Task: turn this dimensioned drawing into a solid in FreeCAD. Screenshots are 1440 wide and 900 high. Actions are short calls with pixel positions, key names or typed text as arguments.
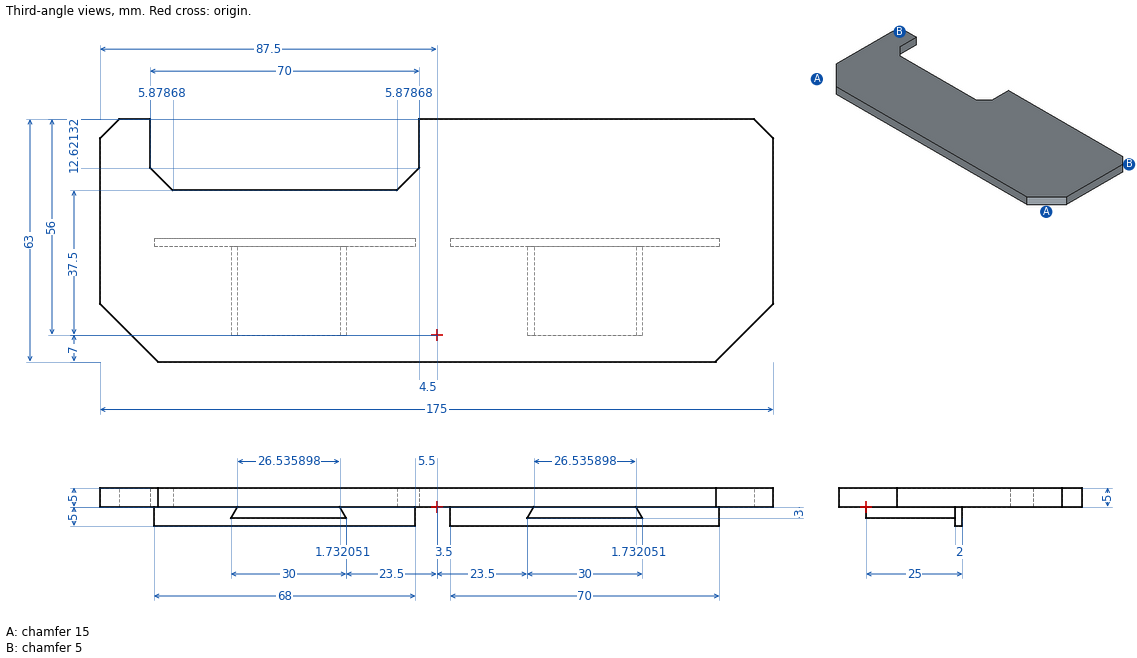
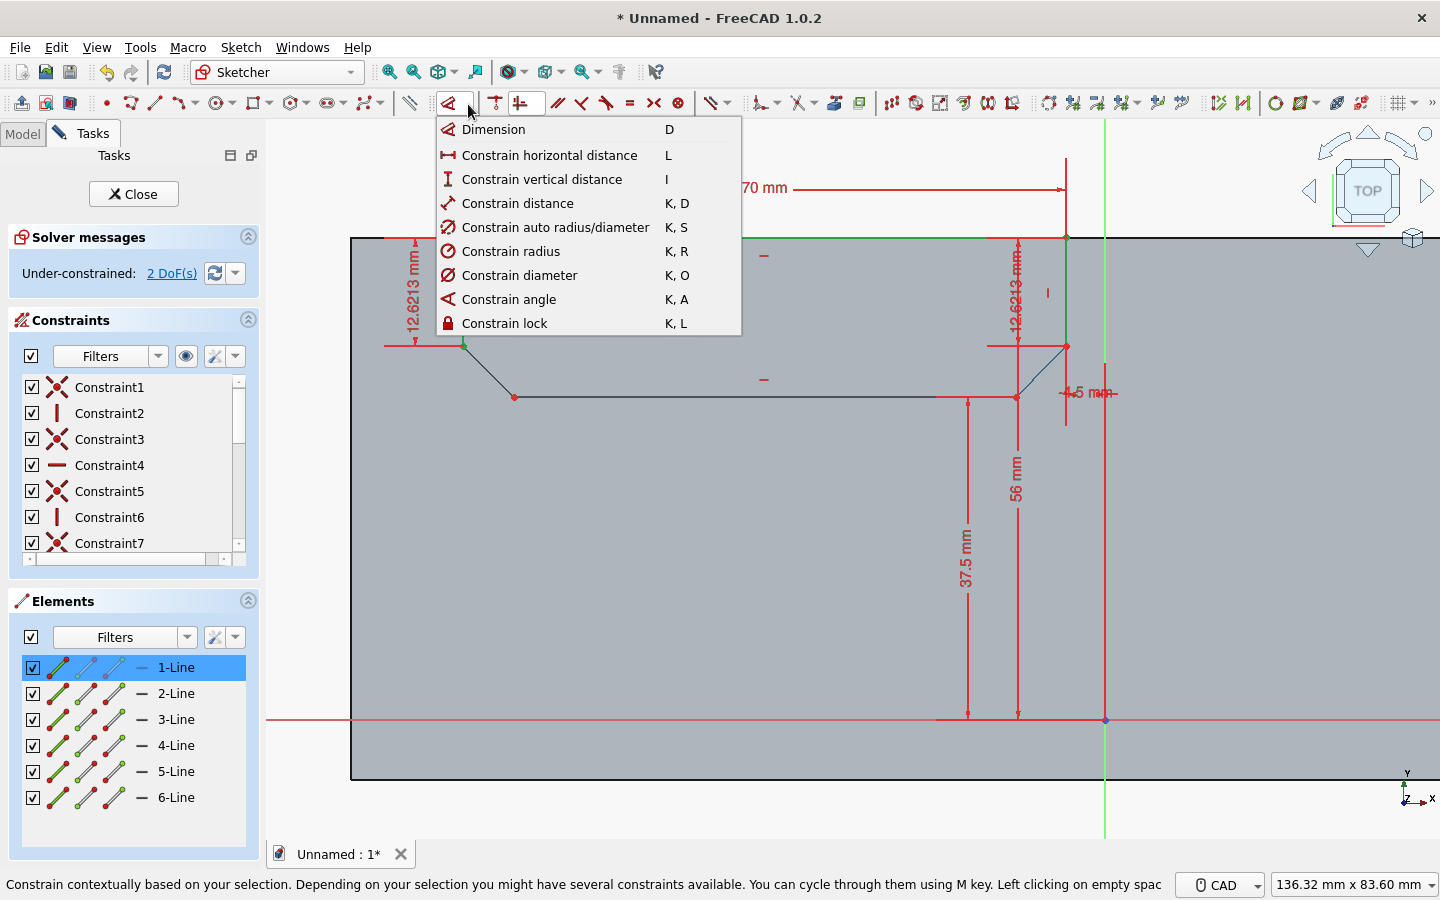
click(589, 155)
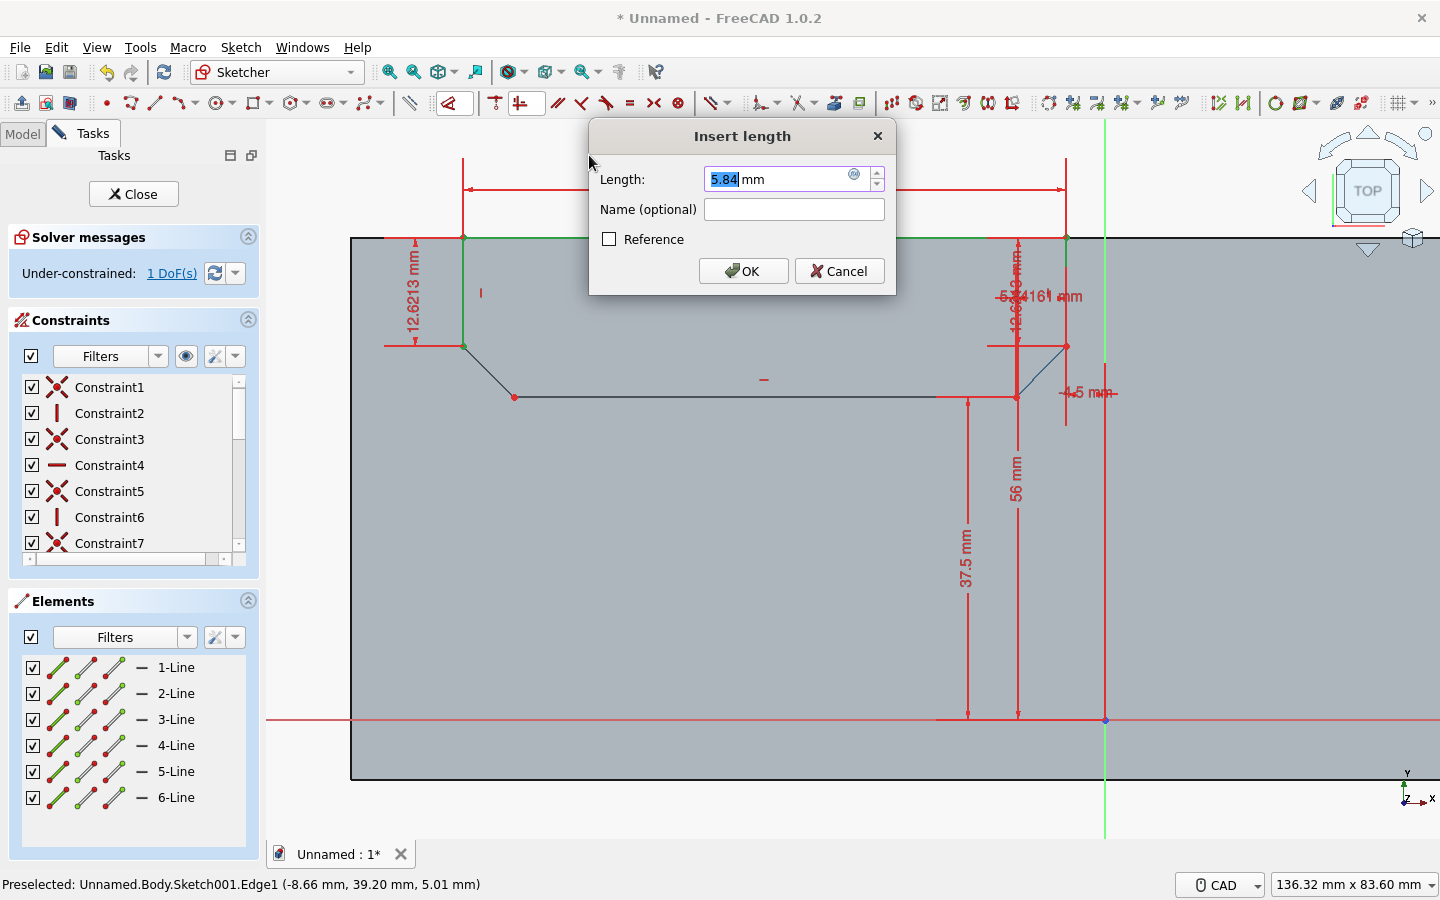
text(5.87868)
key(Return)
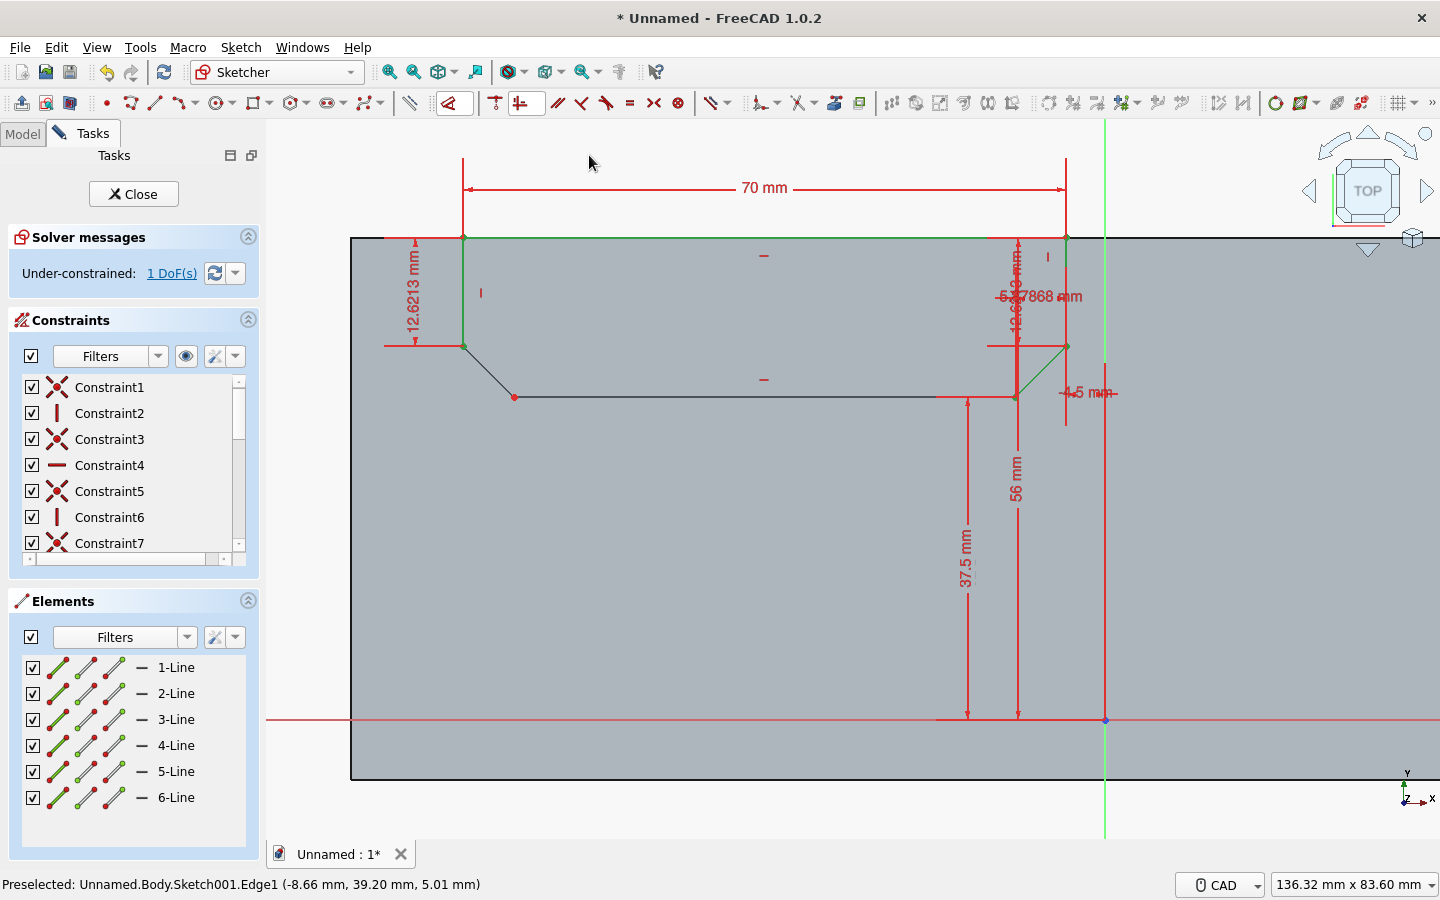
click(479, 362)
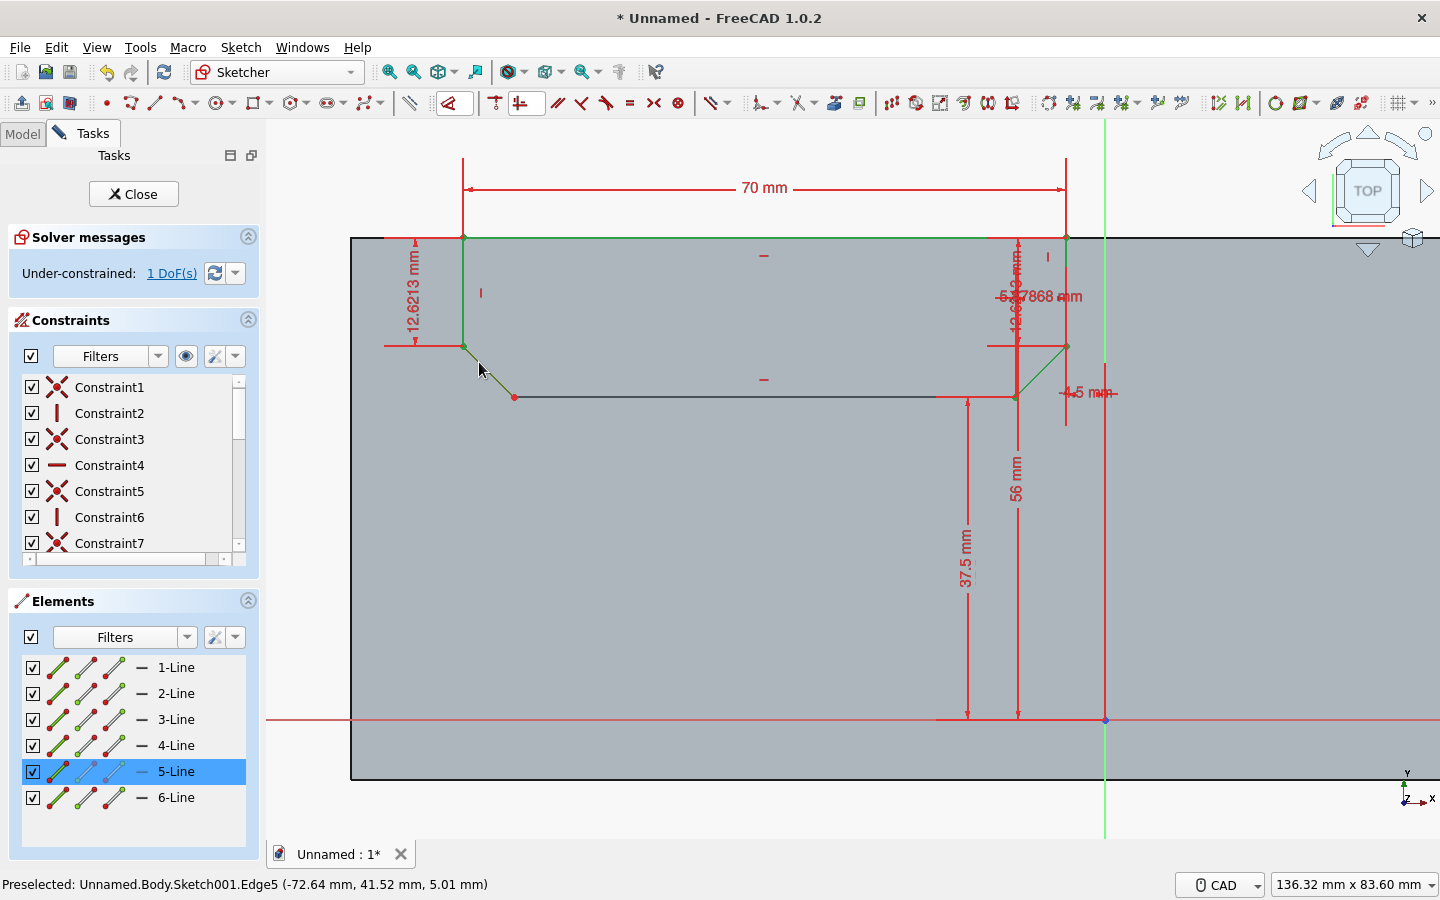
key(l)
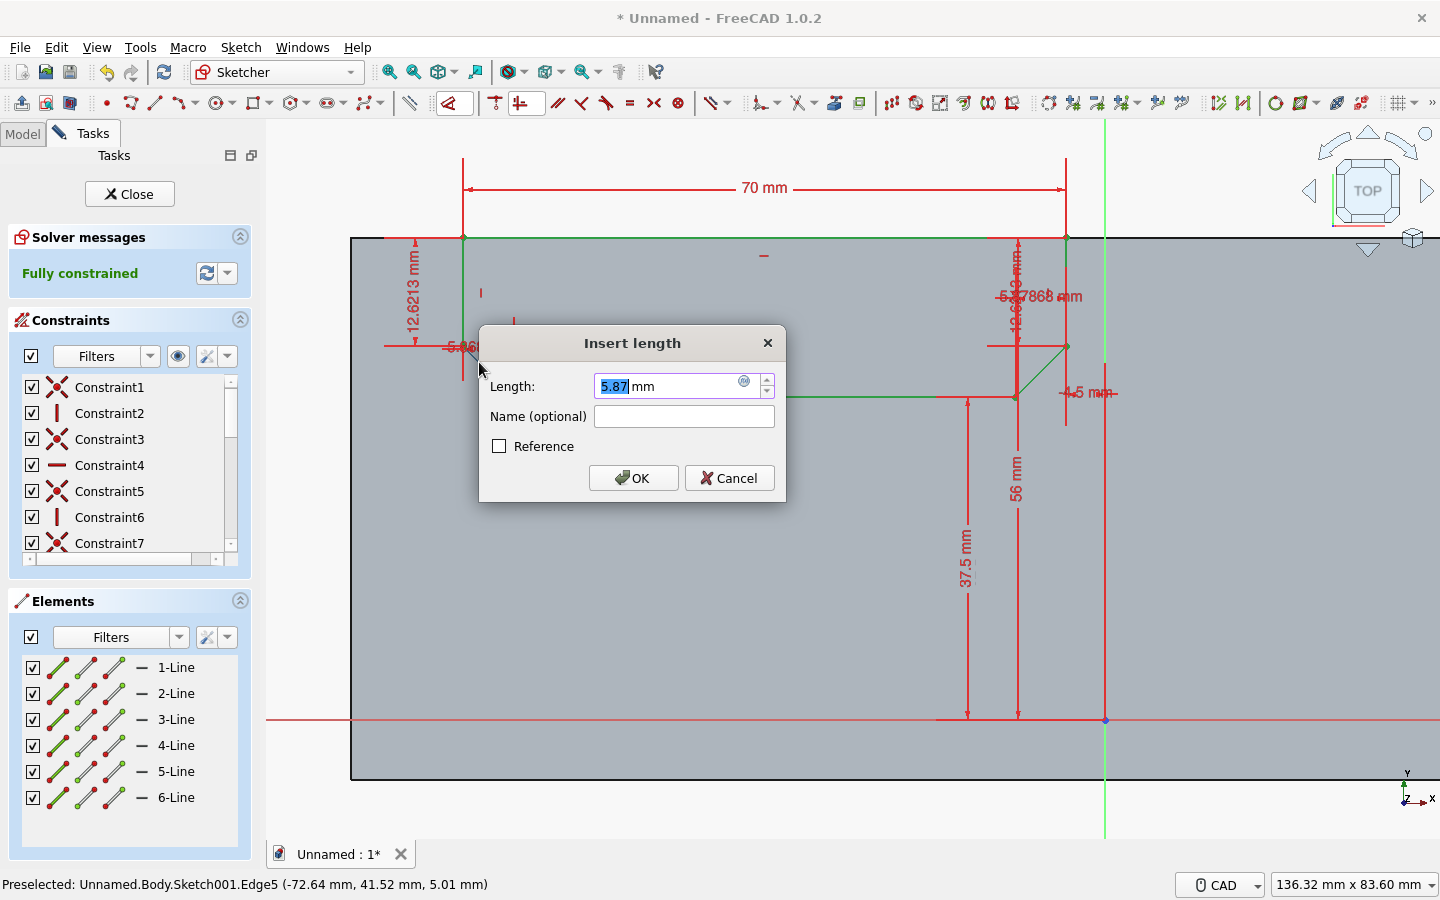
text(5.87868)
key(Return)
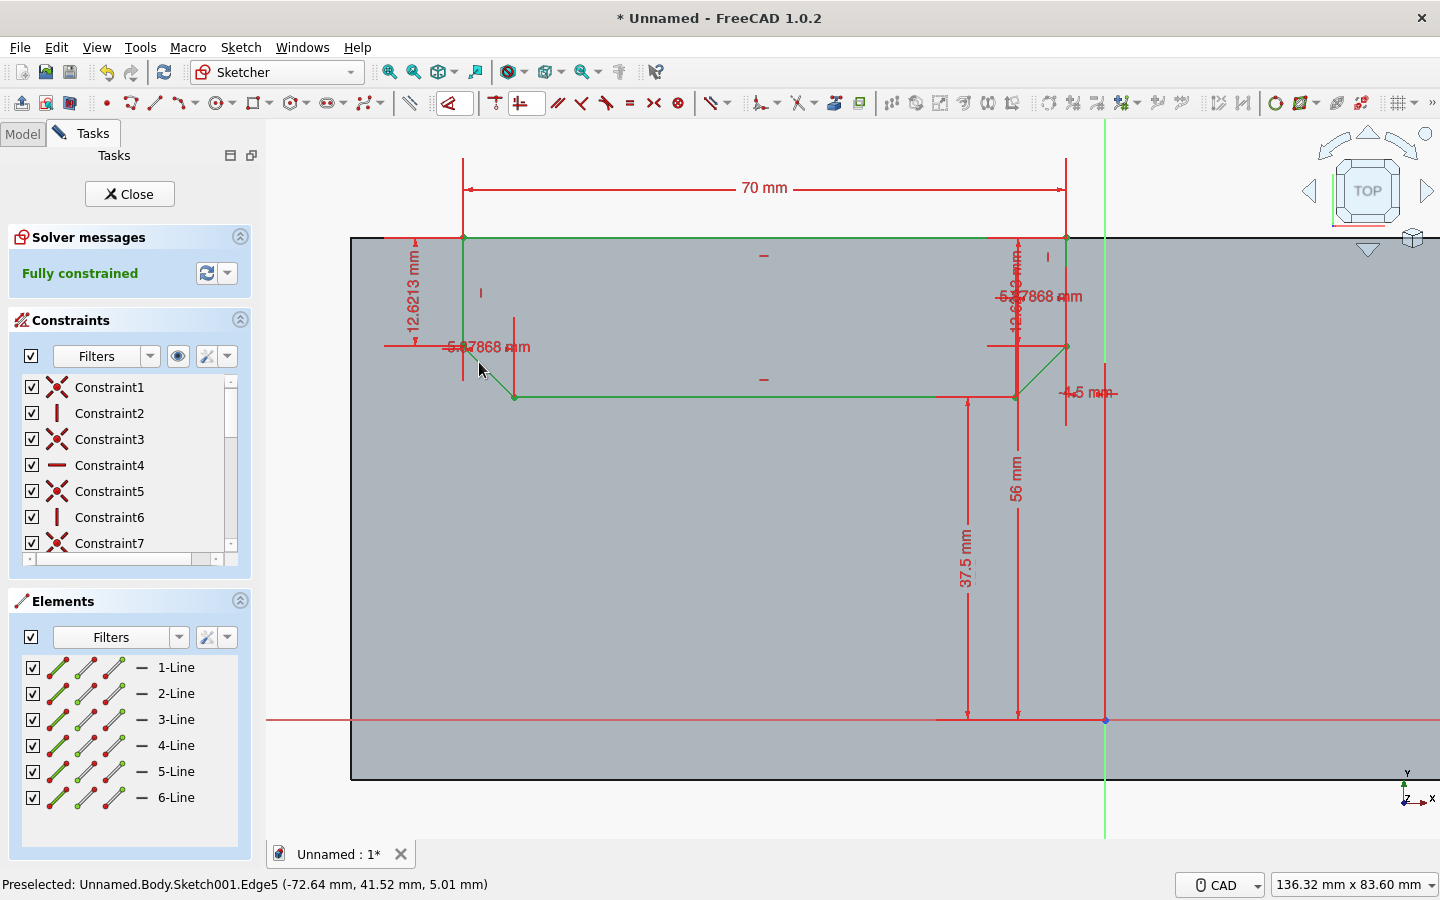
click(130, 194)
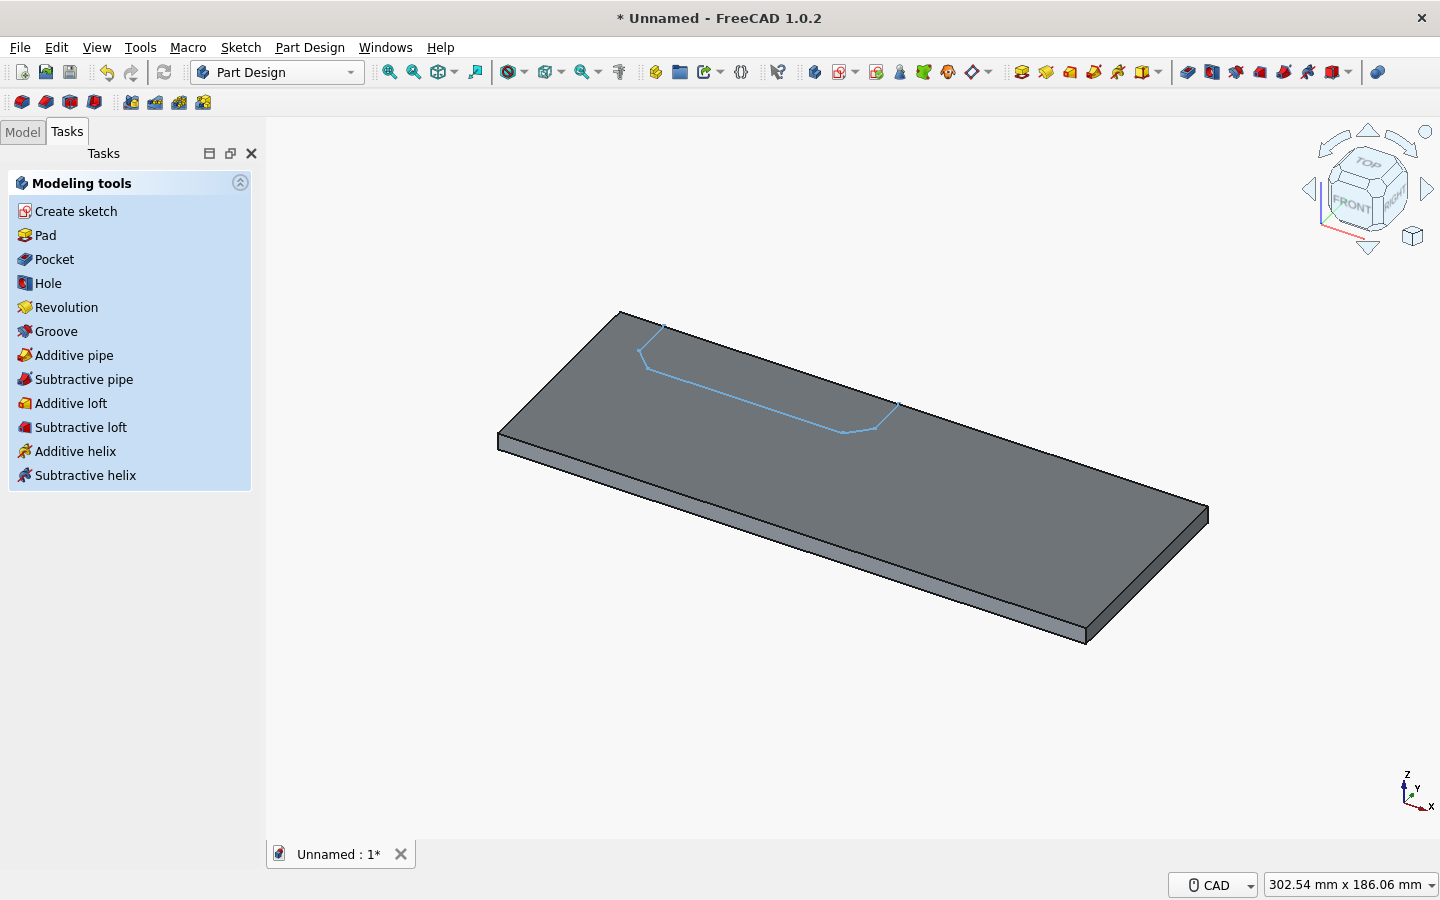
click(1188, 72)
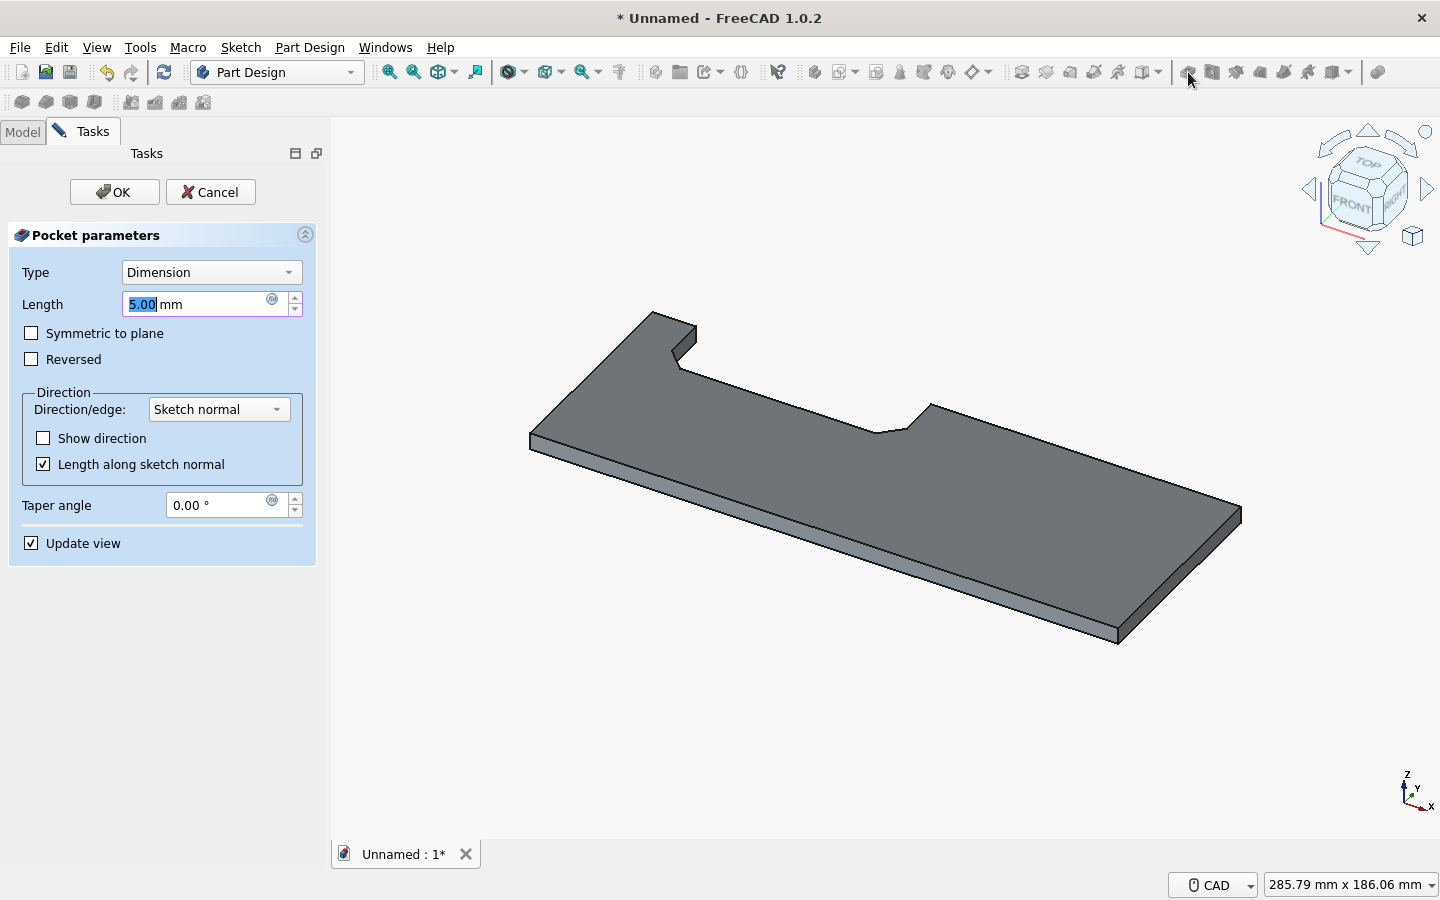
text(5)
key(Tab)